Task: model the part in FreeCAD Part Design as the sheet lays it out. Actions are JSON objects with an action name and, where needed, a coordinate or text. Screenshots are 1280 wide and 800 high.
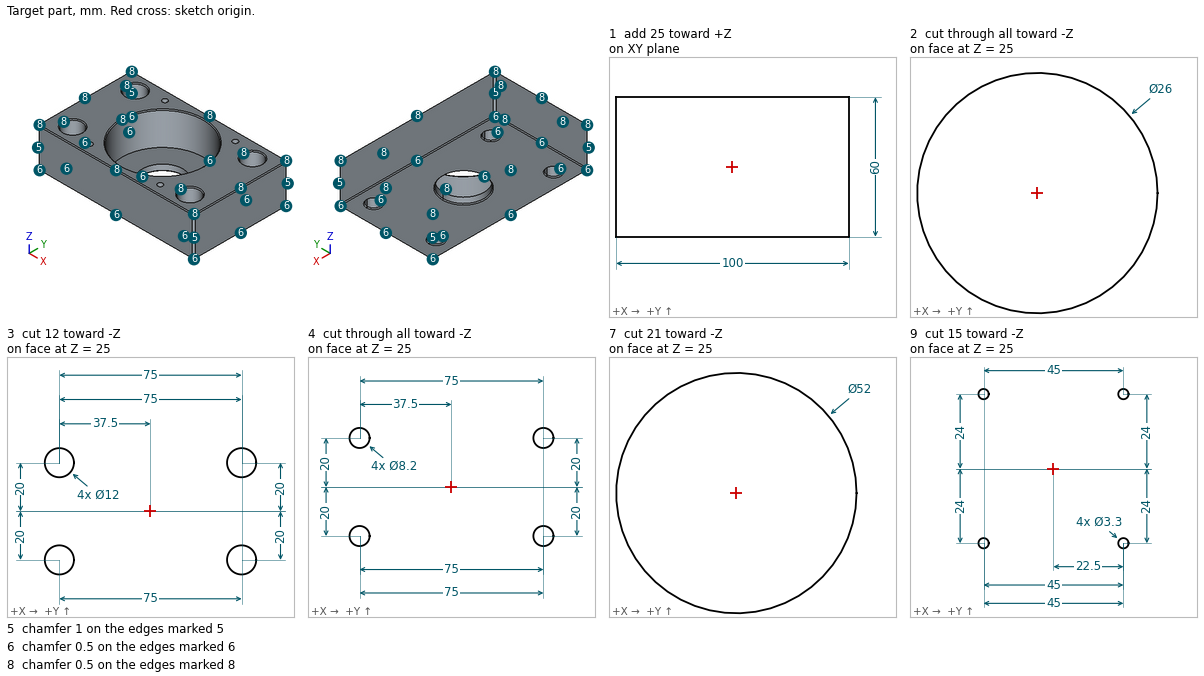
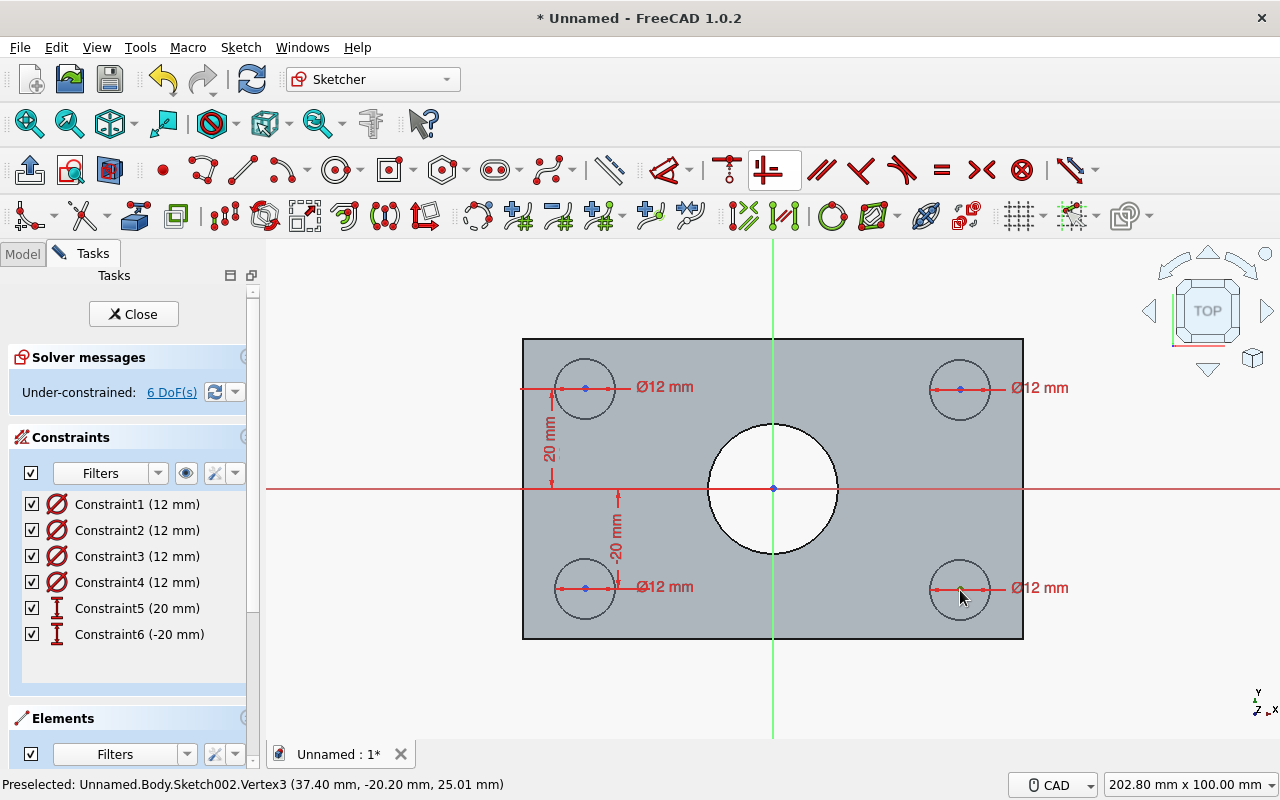
{"action": "key", "text": "i"}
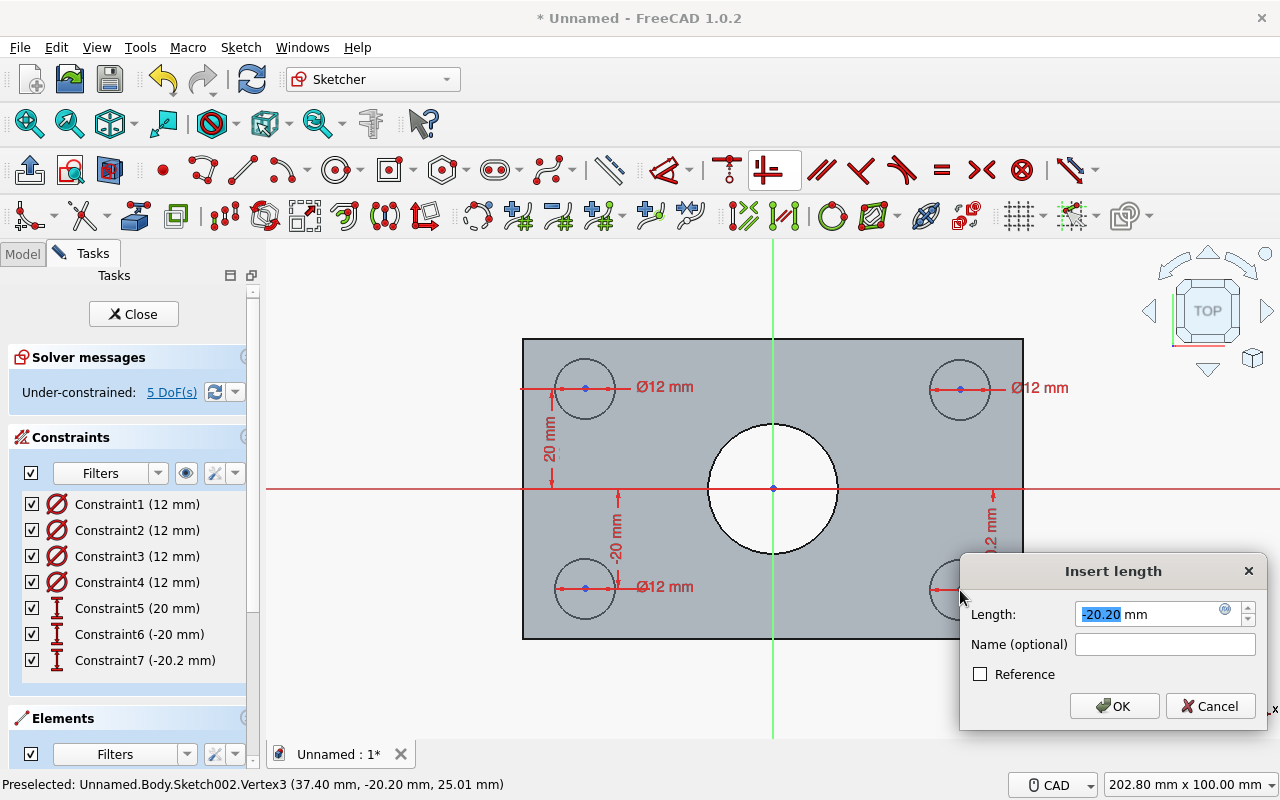
{"action": "type", "text": "-20"}
{"action": "key", "text": "Return"}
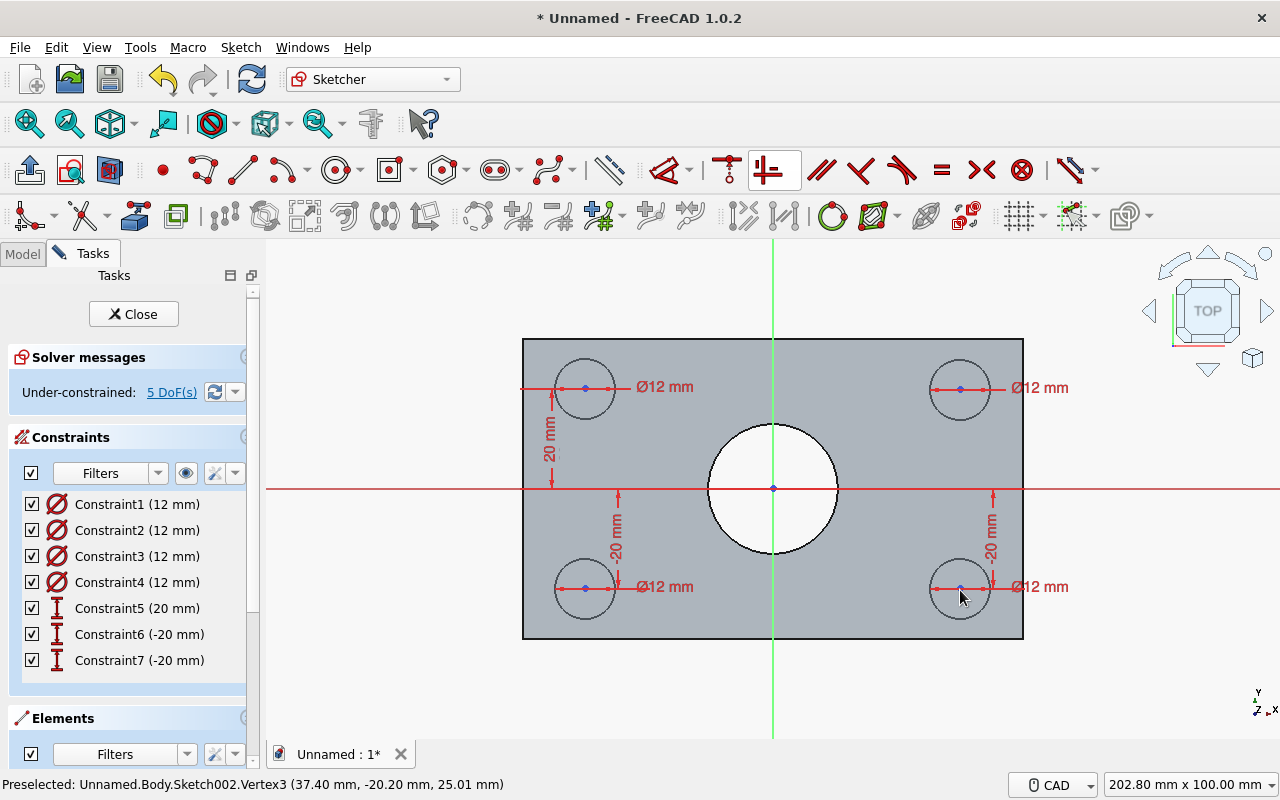
{"action": "left_click", "coordinate": [960, 390]}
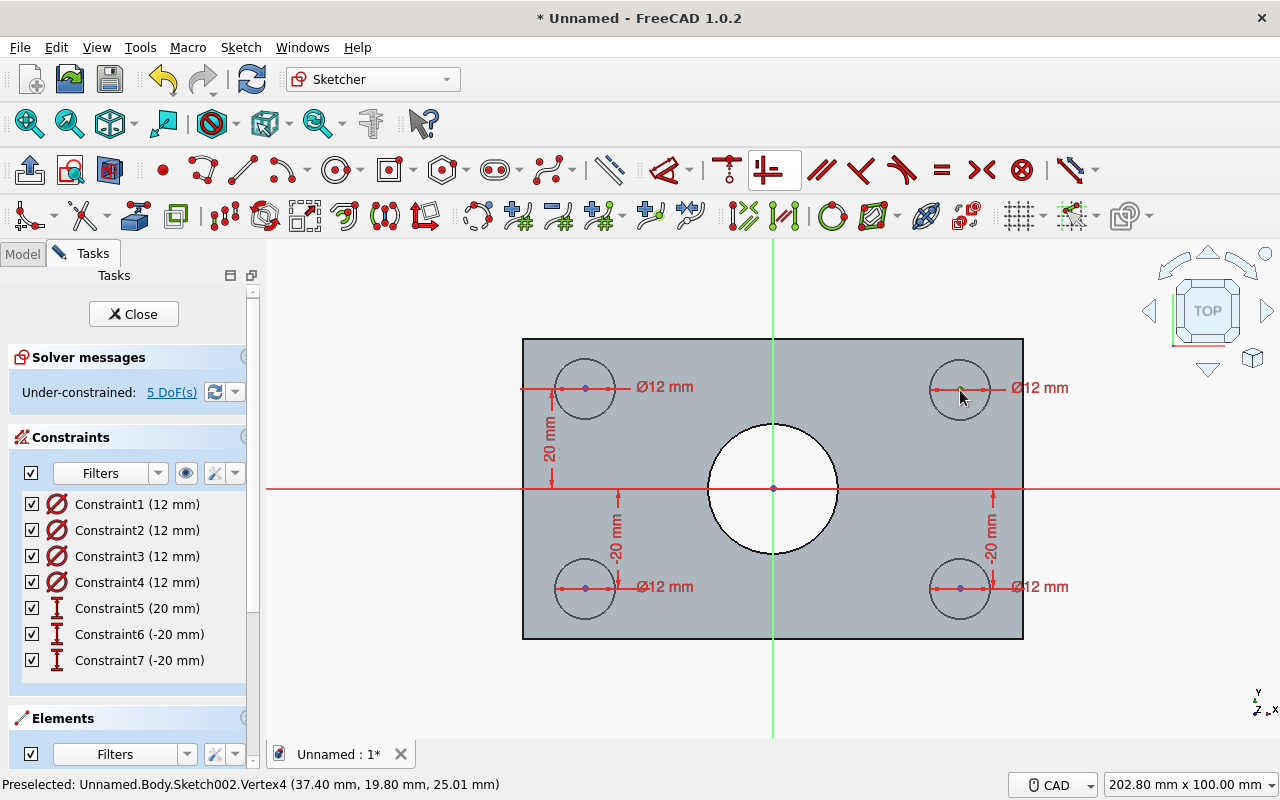
{"action": "key", "text": "i"}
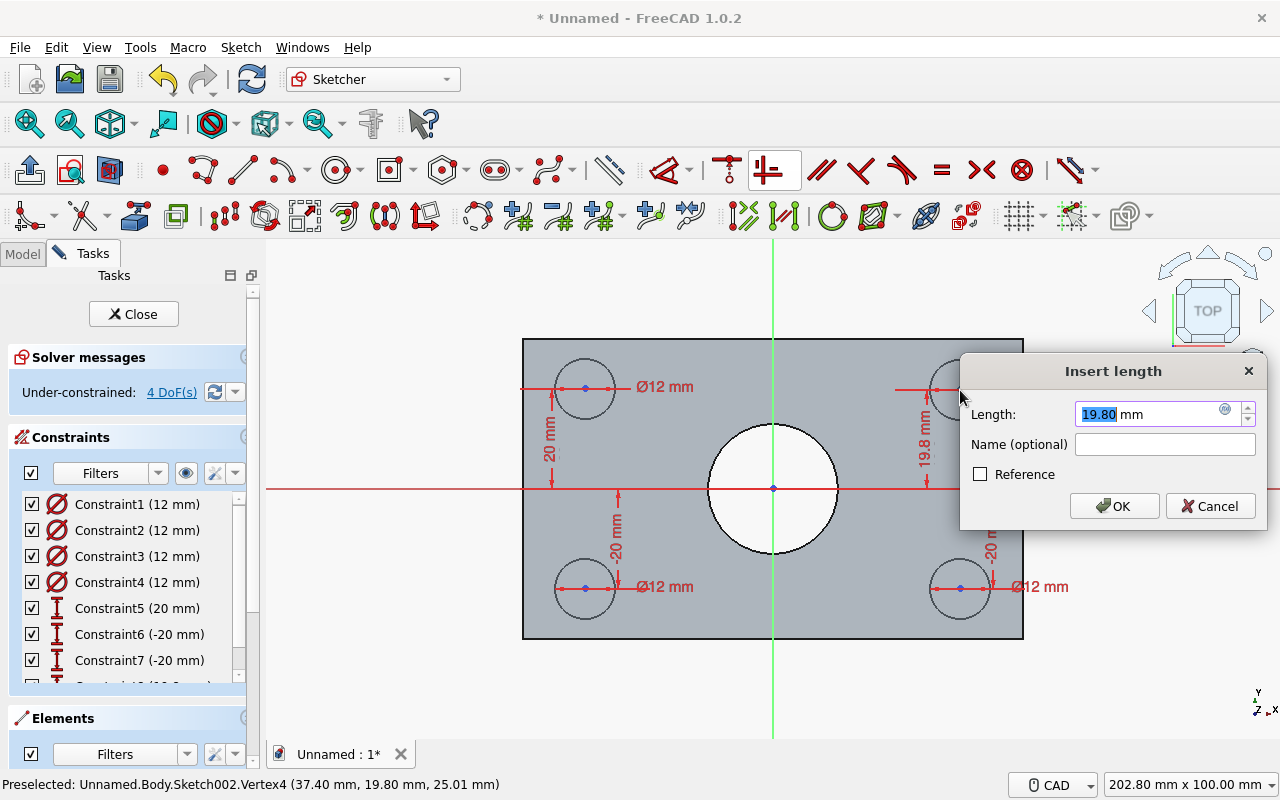
{"action": "type", "text": "20"}
{"action": "key", "text": "Return"}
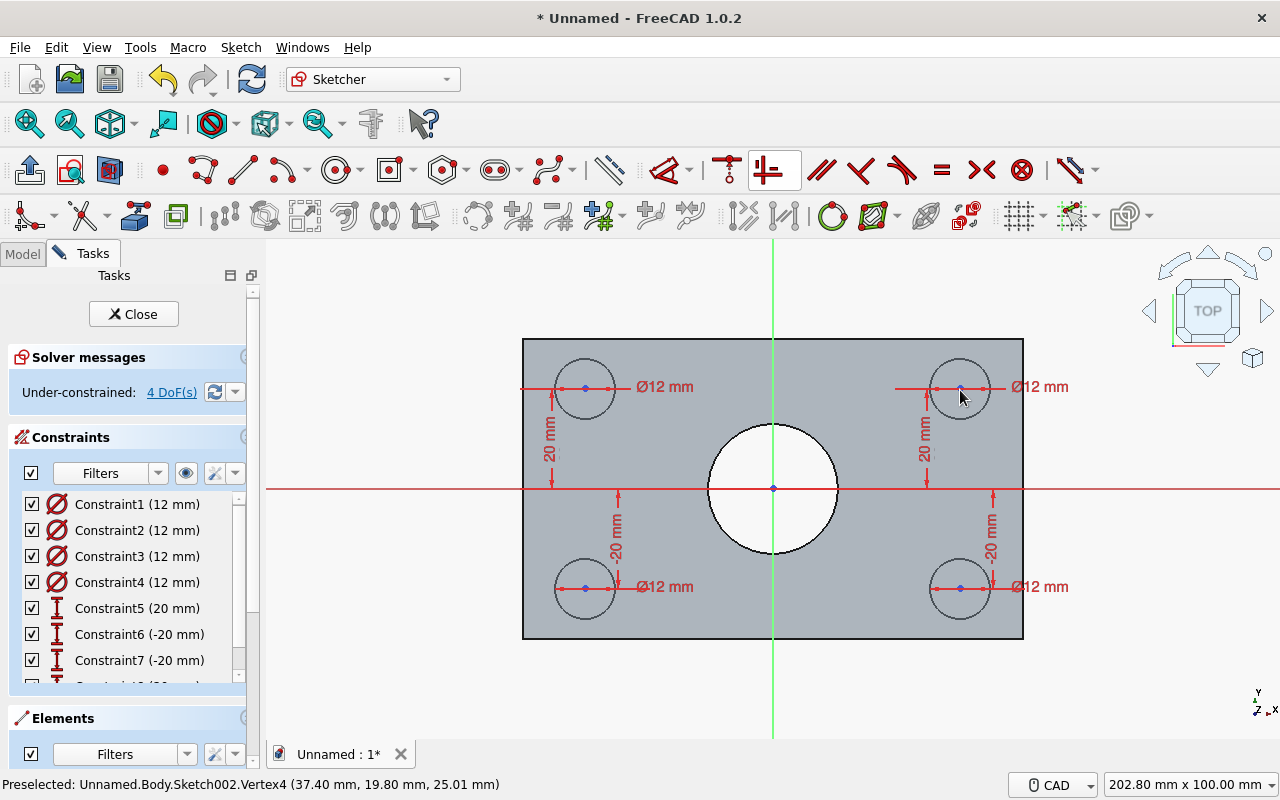
{"action": "left_click", "coordinate": [585, 589]}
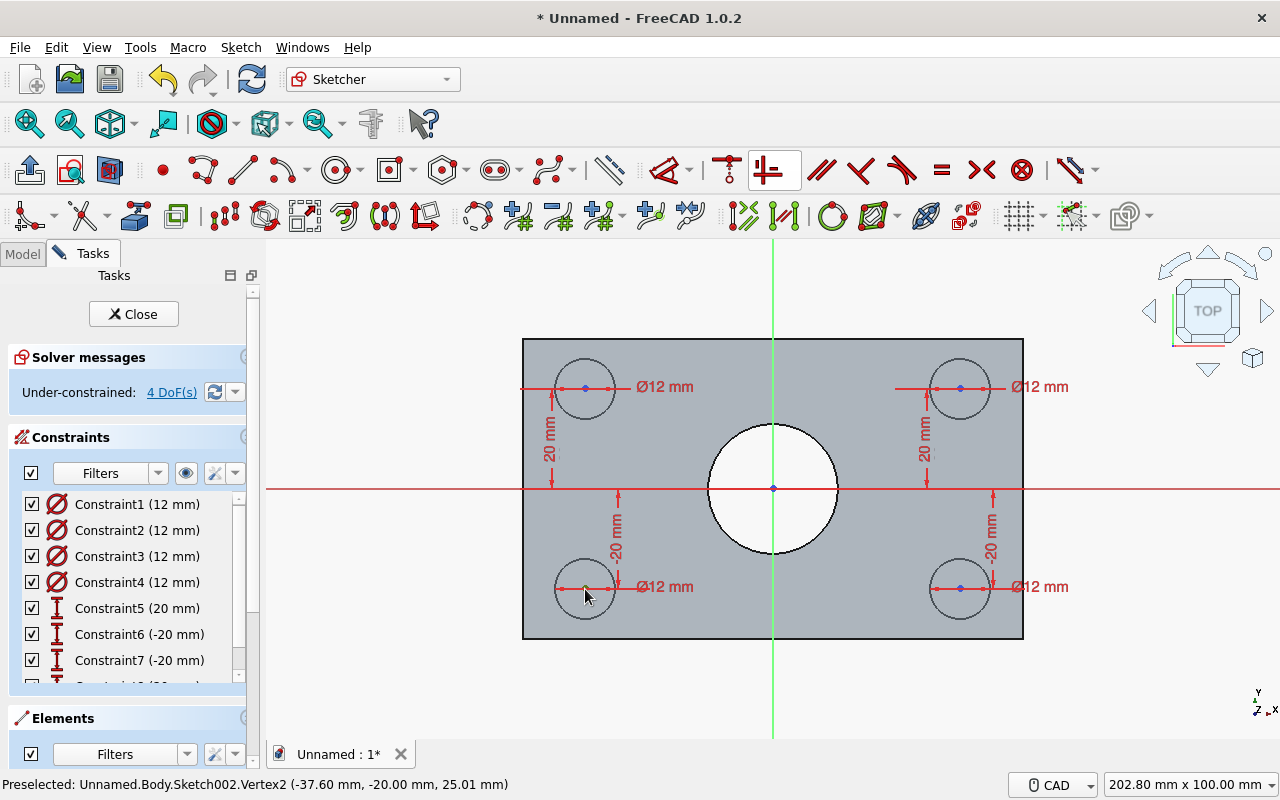
{"action": "left_click", "coordinate": [960, 589]}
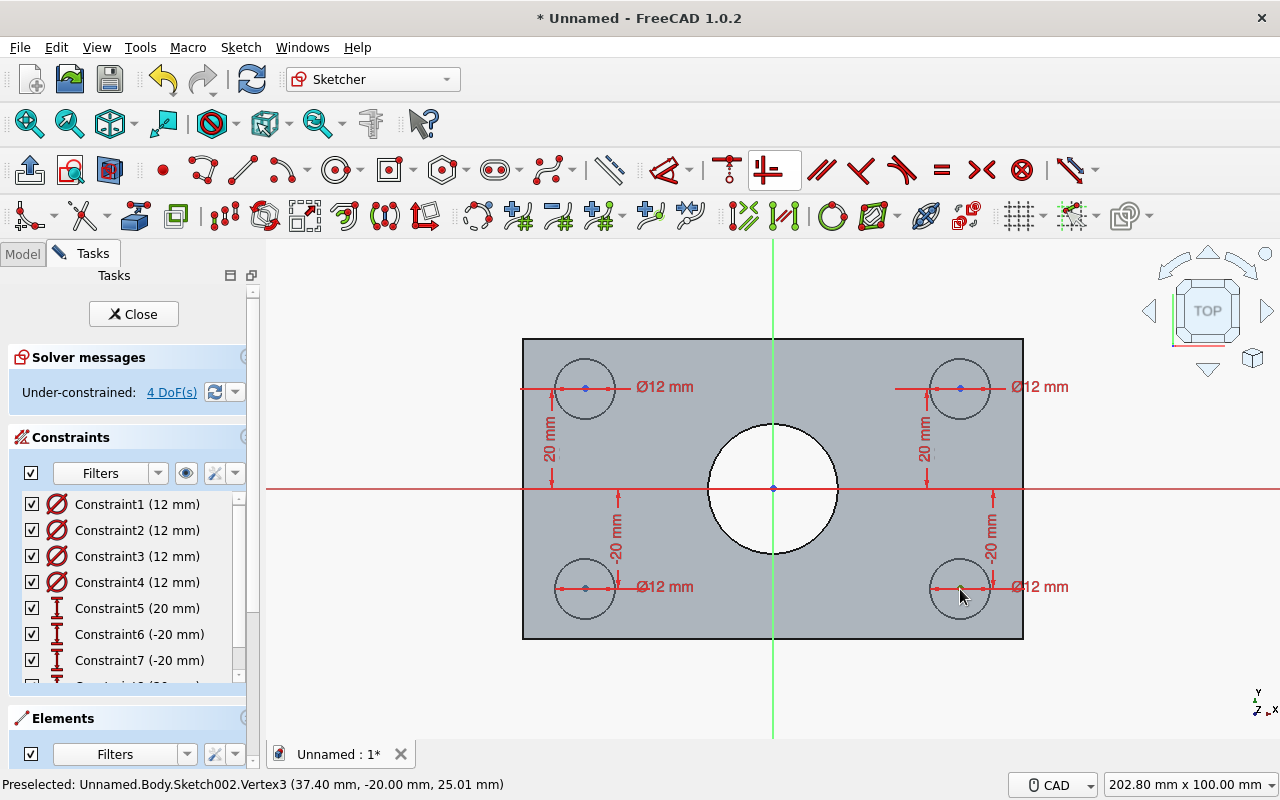
{"action": "key", "text": "l"}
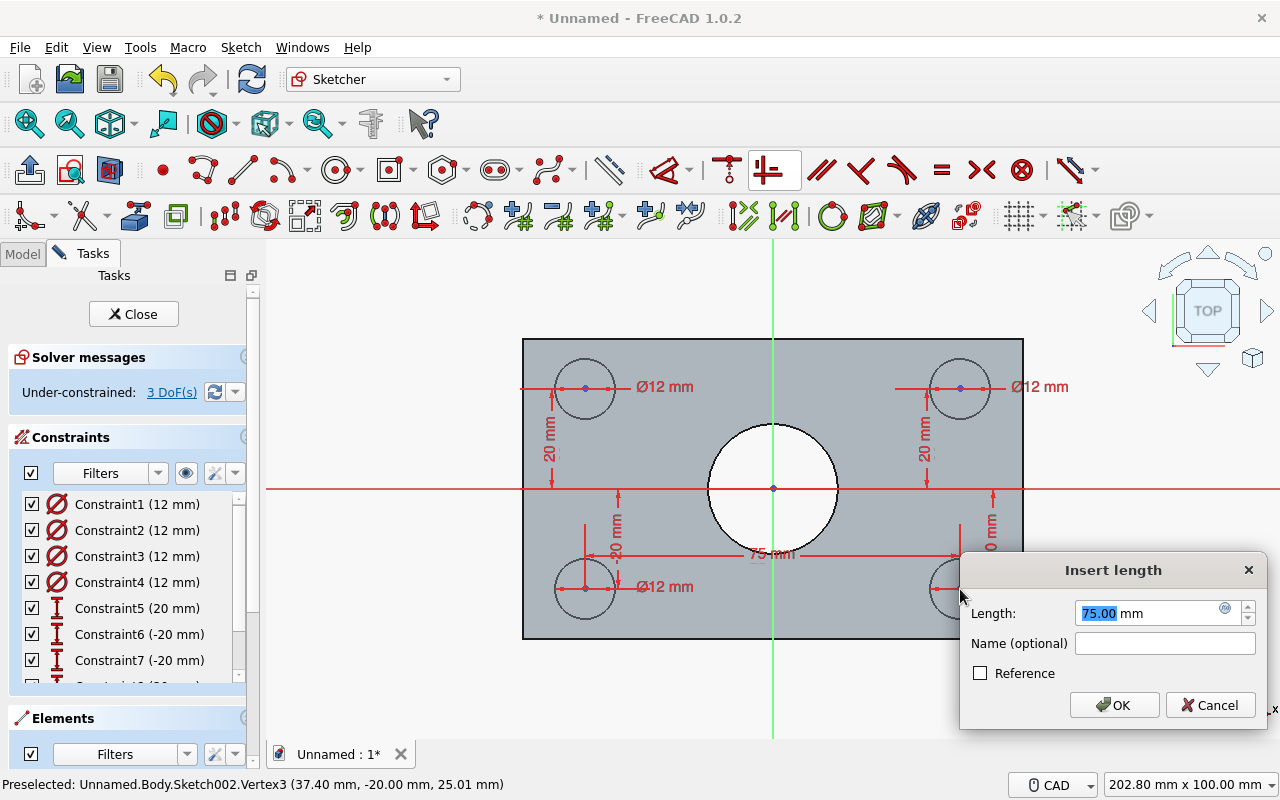
{"action": "type", "text": "75"}
{"action": "key", "text": "Return"}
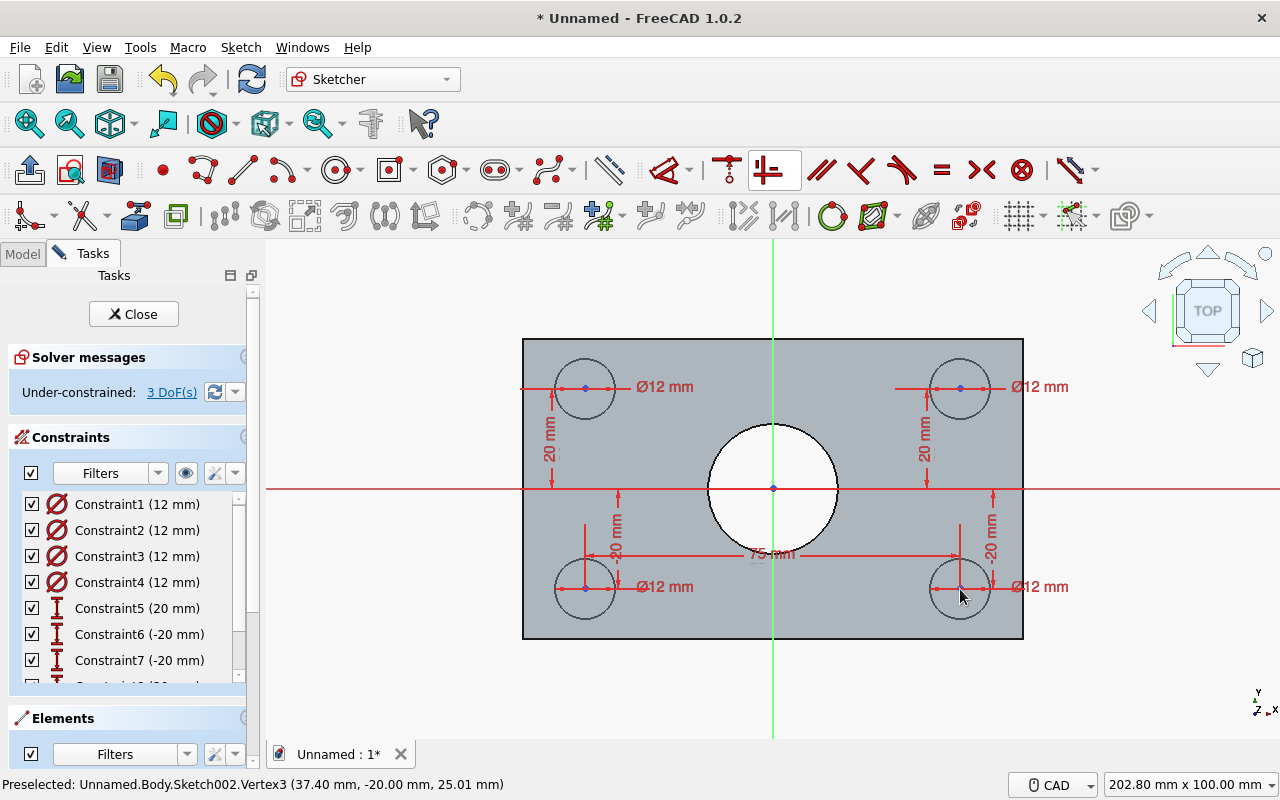
{"action": "left_click", "coordinate": [585, 389]}